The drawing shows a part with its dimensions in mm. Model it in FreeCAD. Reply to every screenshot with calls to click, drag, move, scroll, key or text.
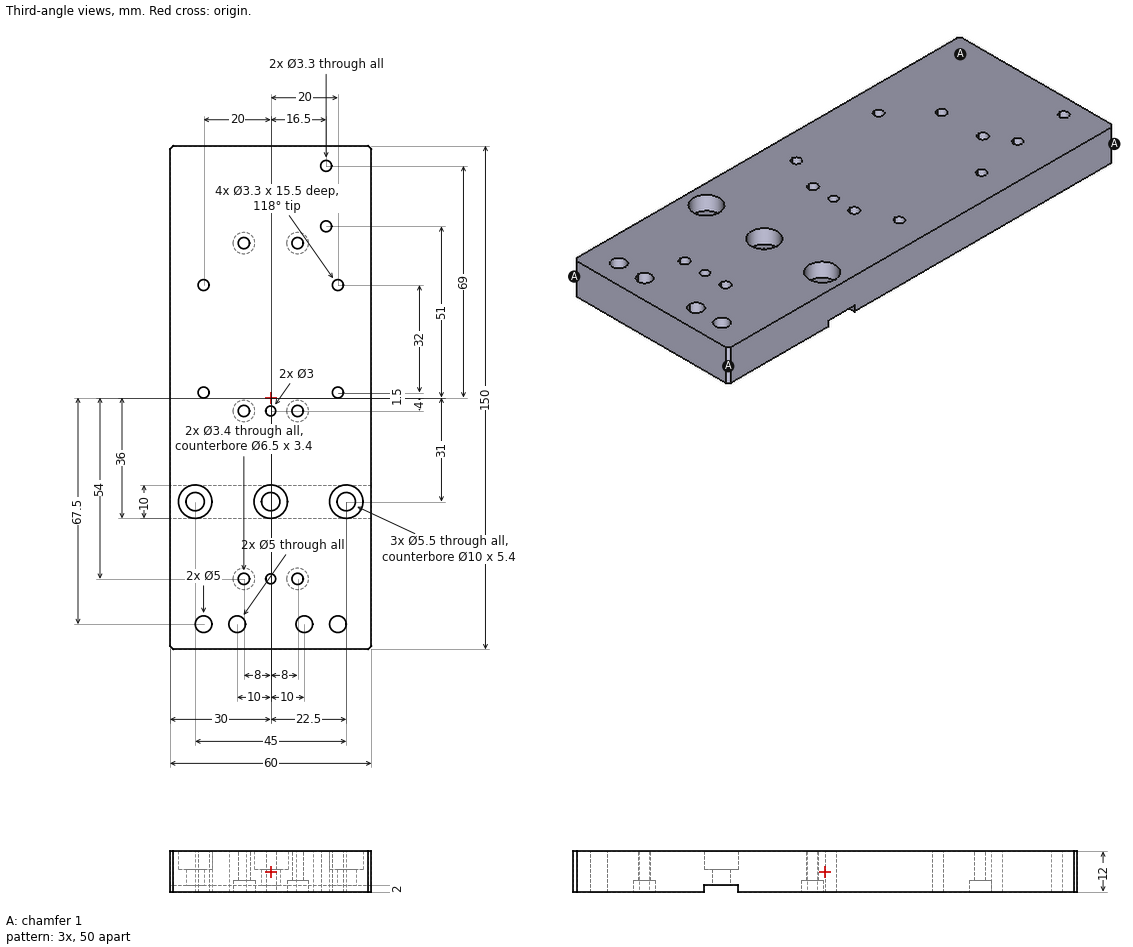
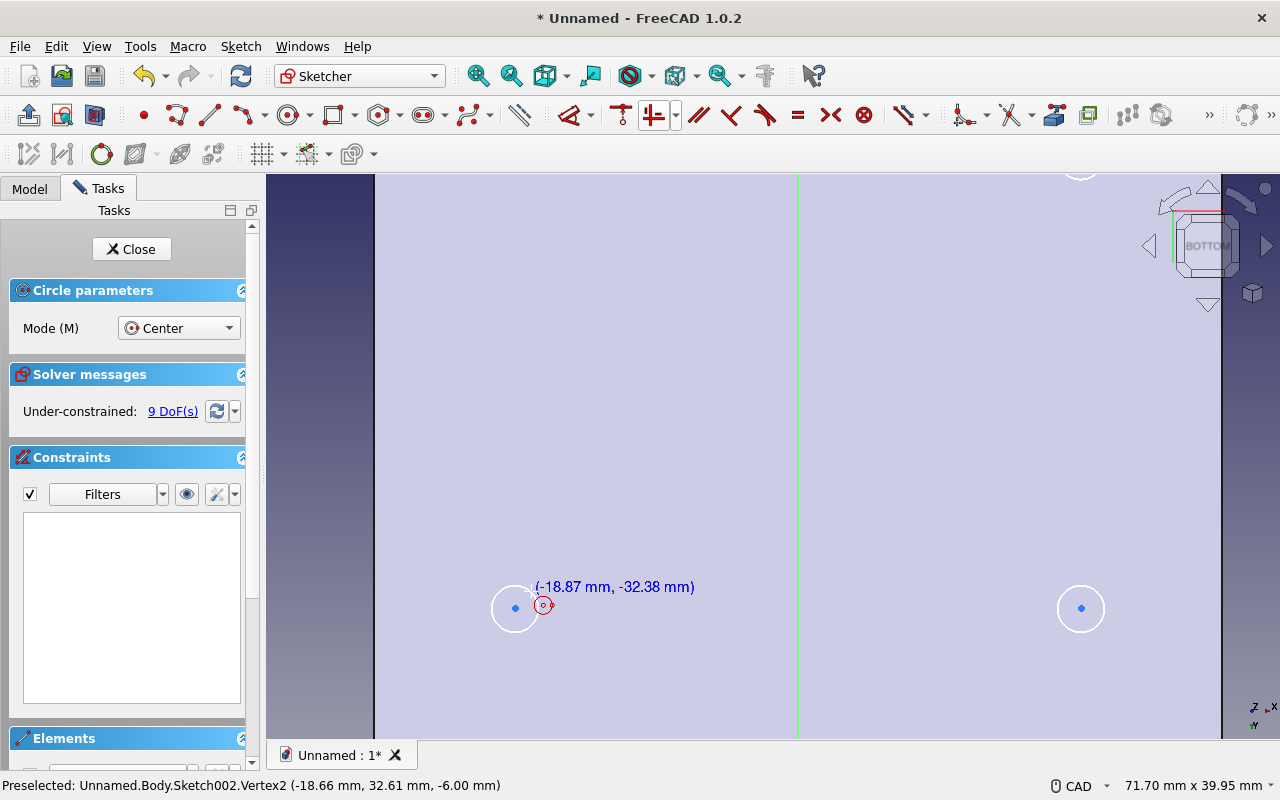
scroll(515, 609, down, 2)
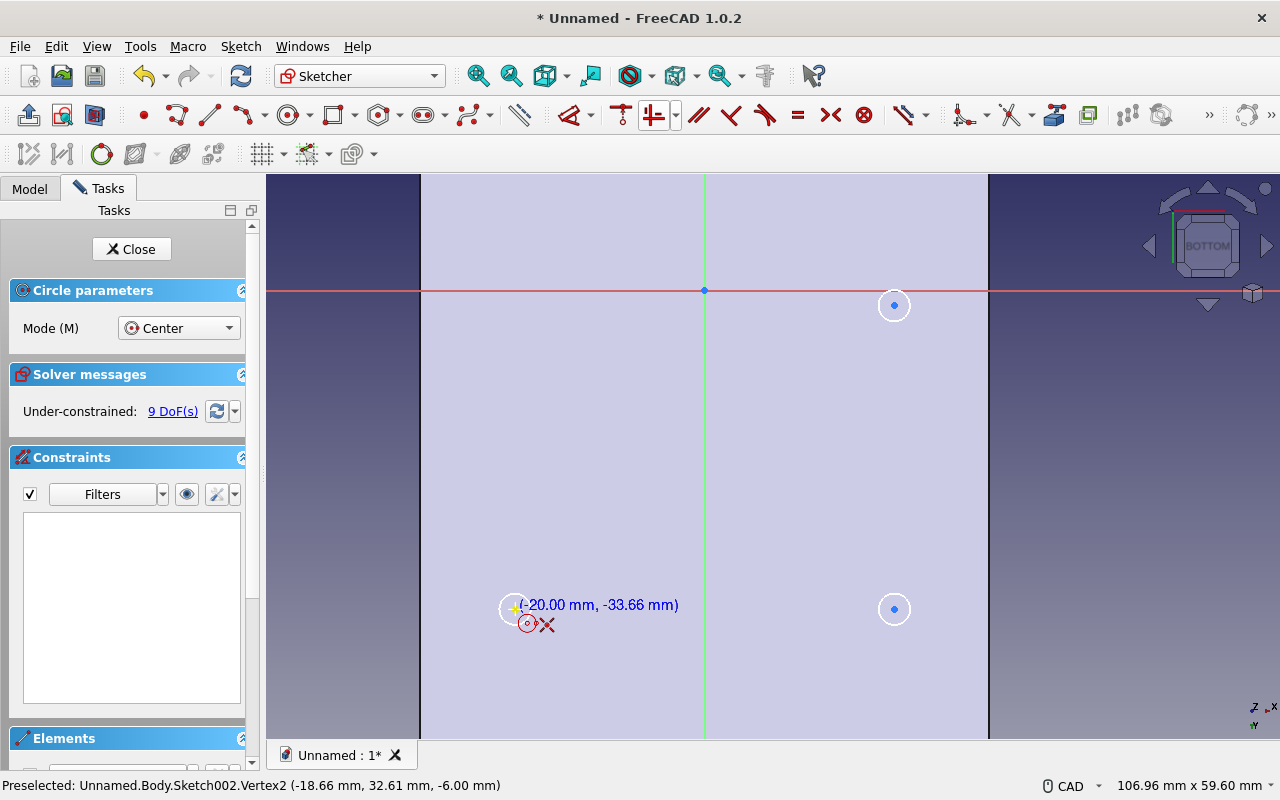
scroll(515, 305, up, 2)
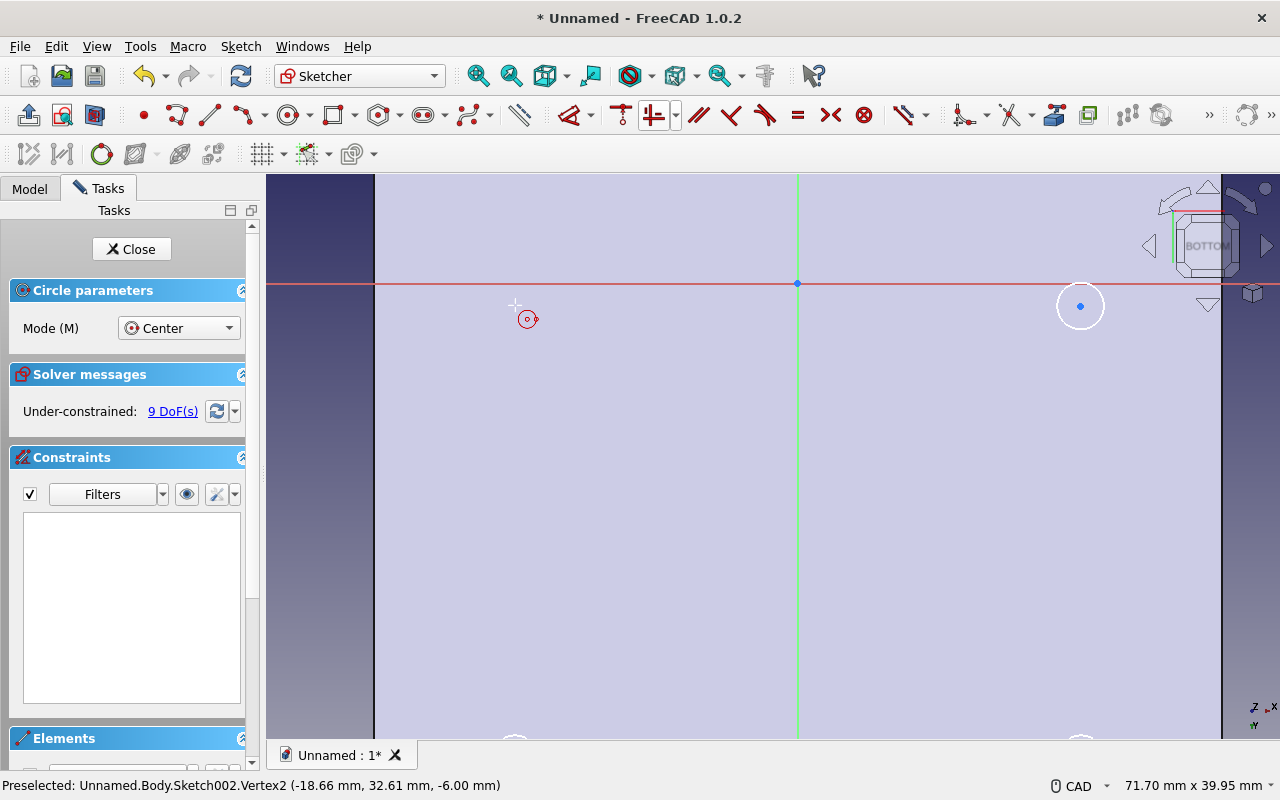
click(515, 305)
click(531, 321)
key(Escape)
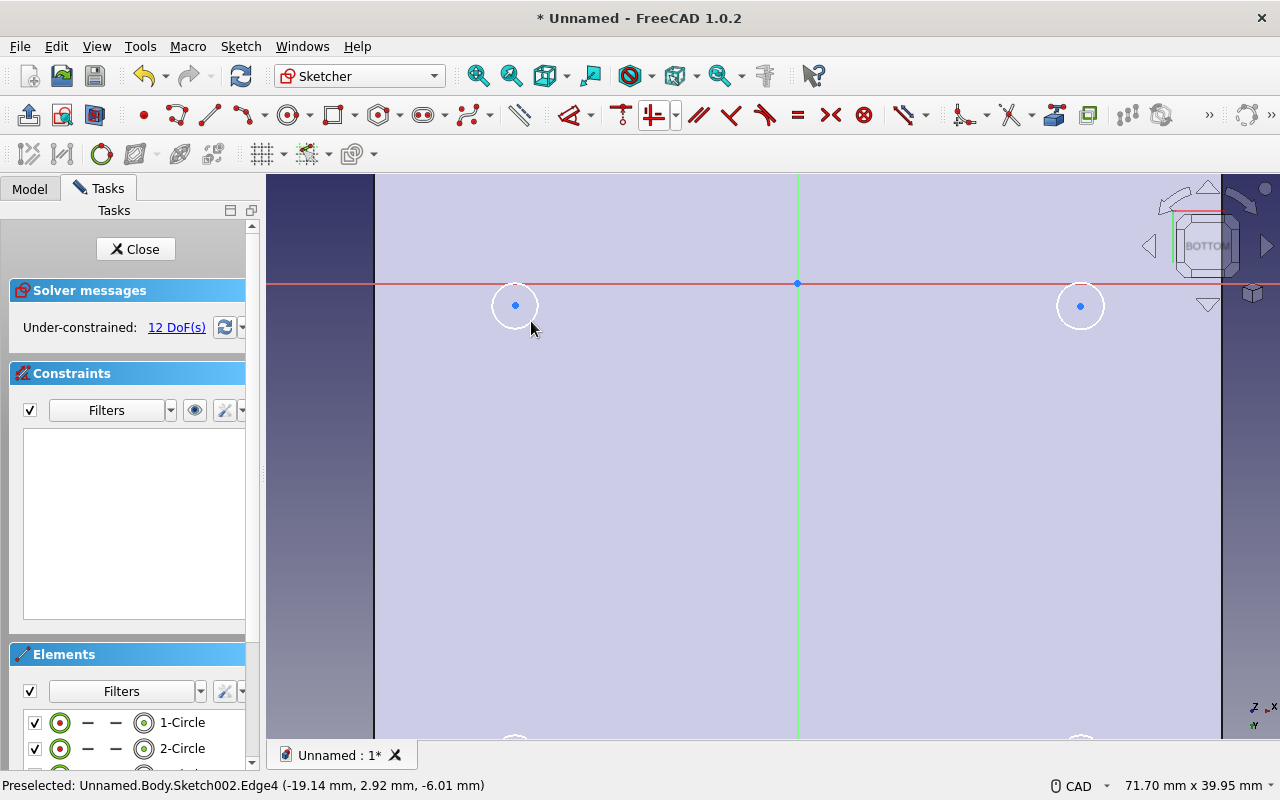
scroll(515, 304, down, 2)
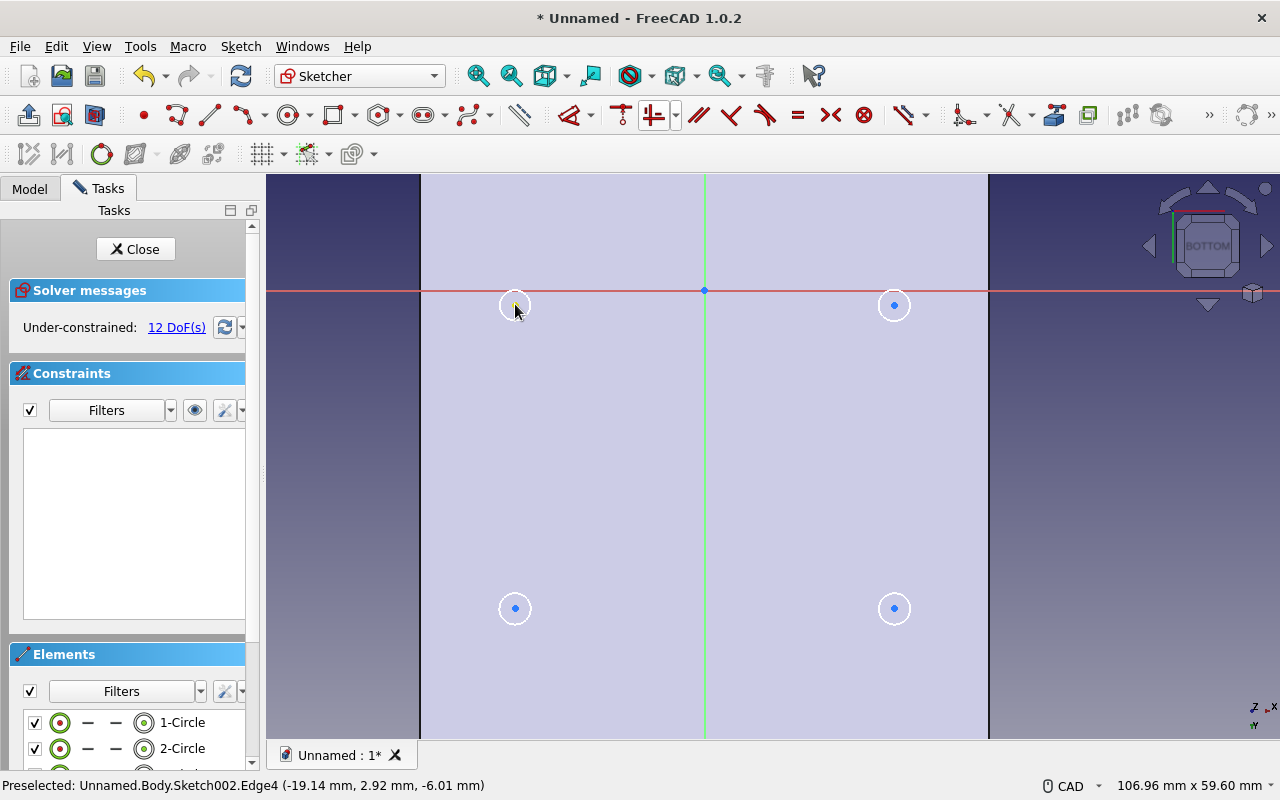
click(906, 598)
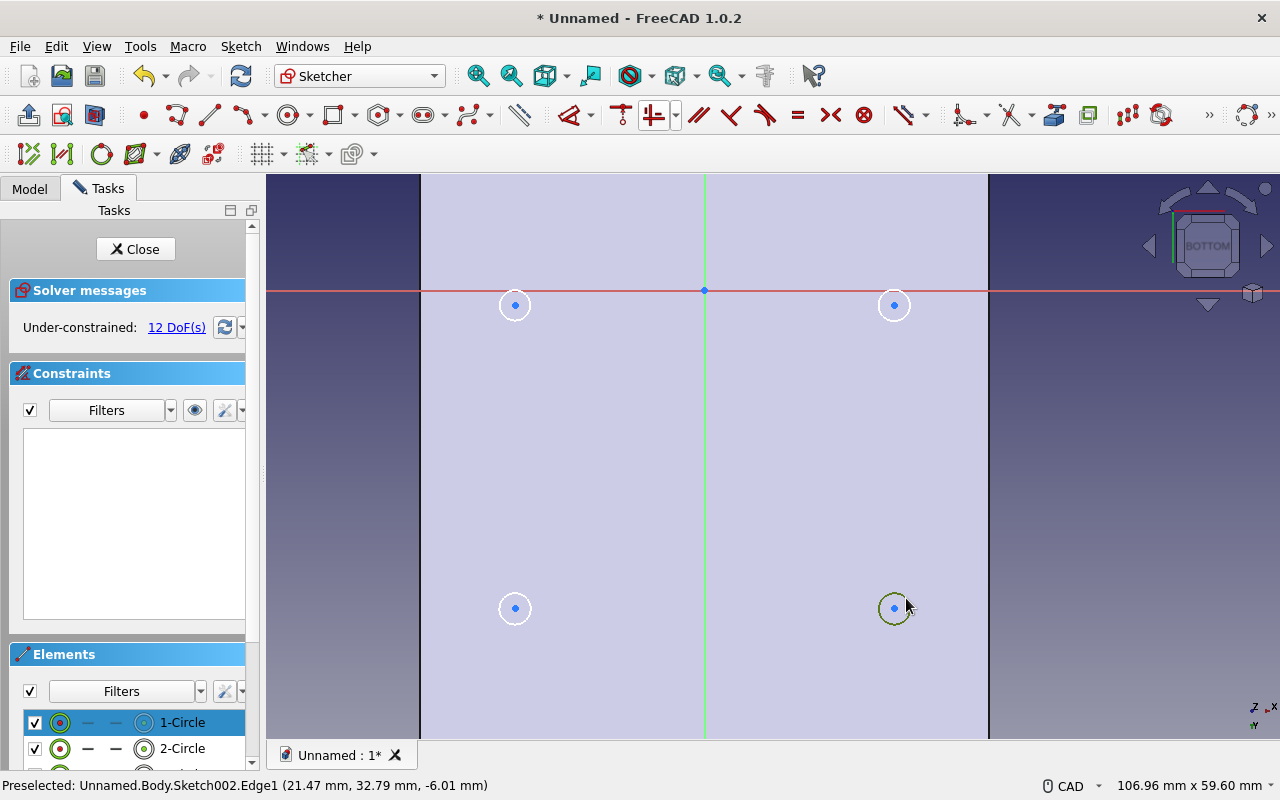
click(905, 294)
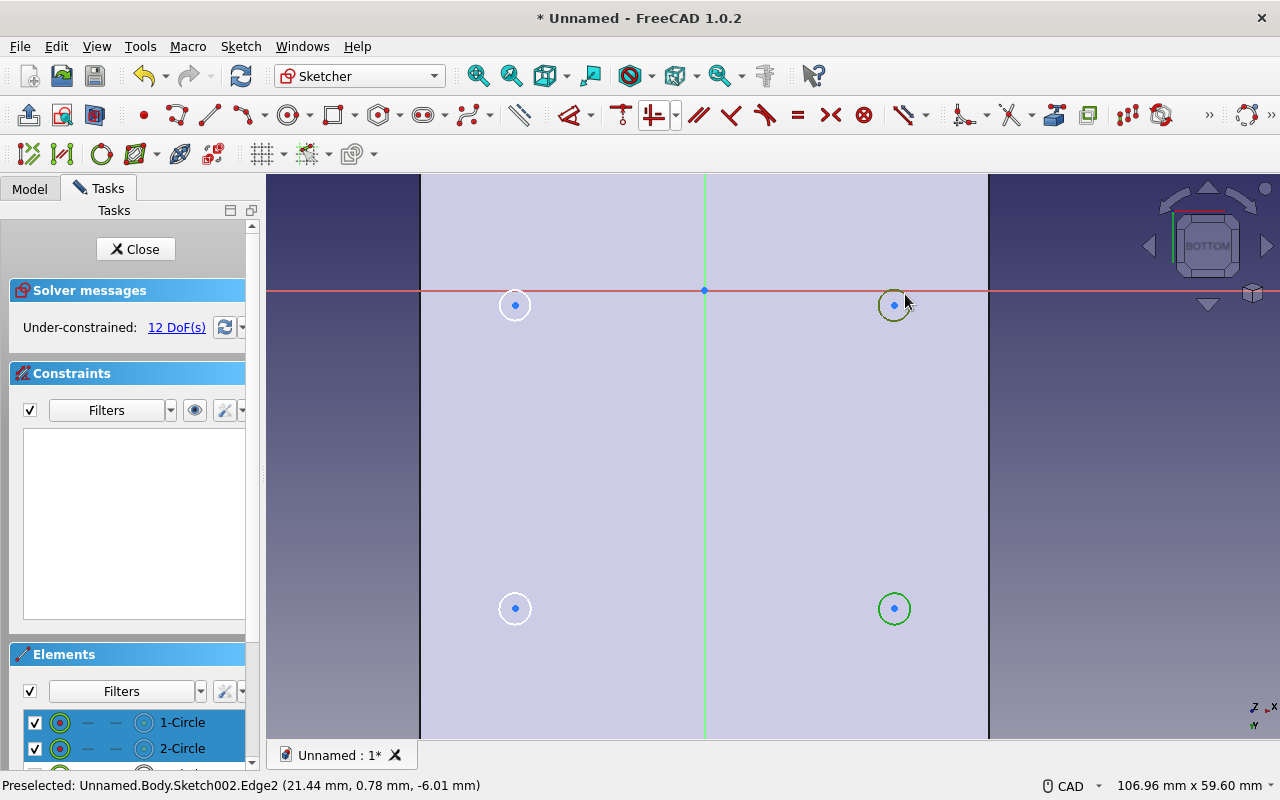
click(526, 598)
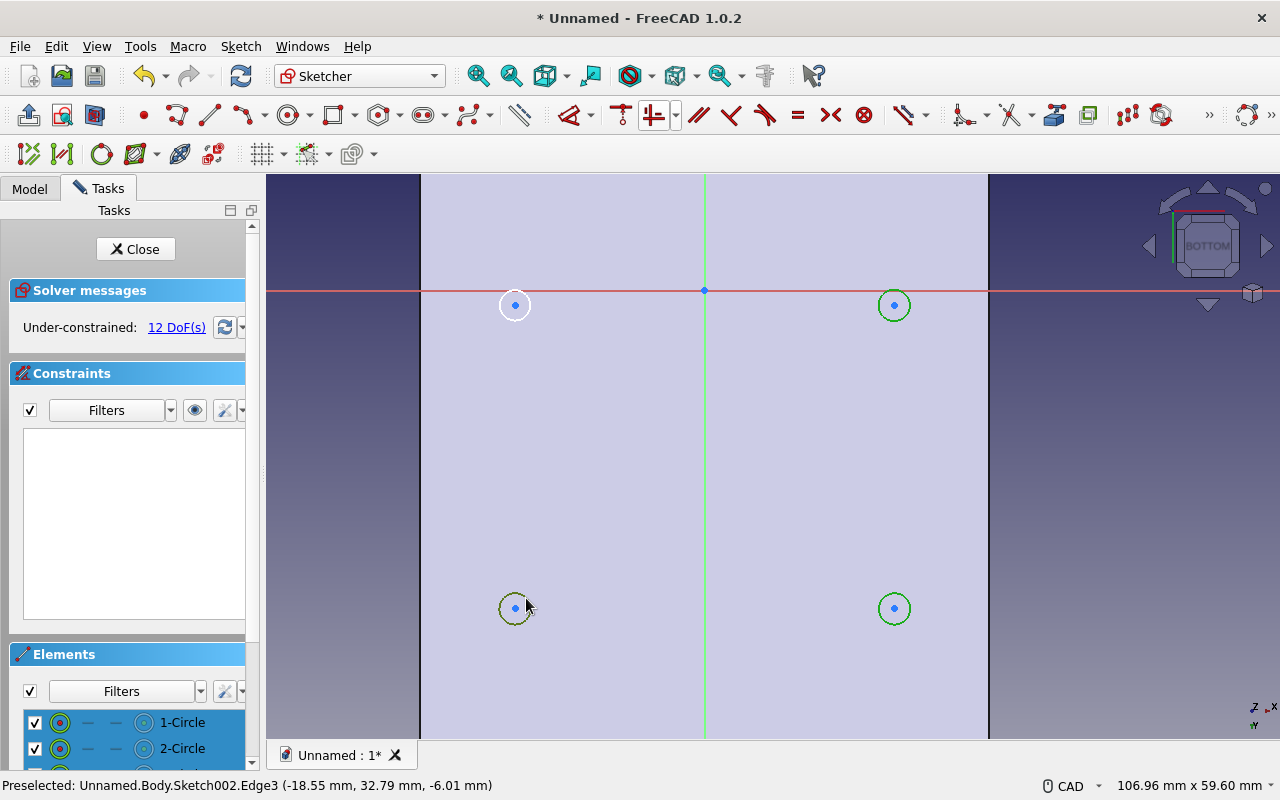
click(504, 316)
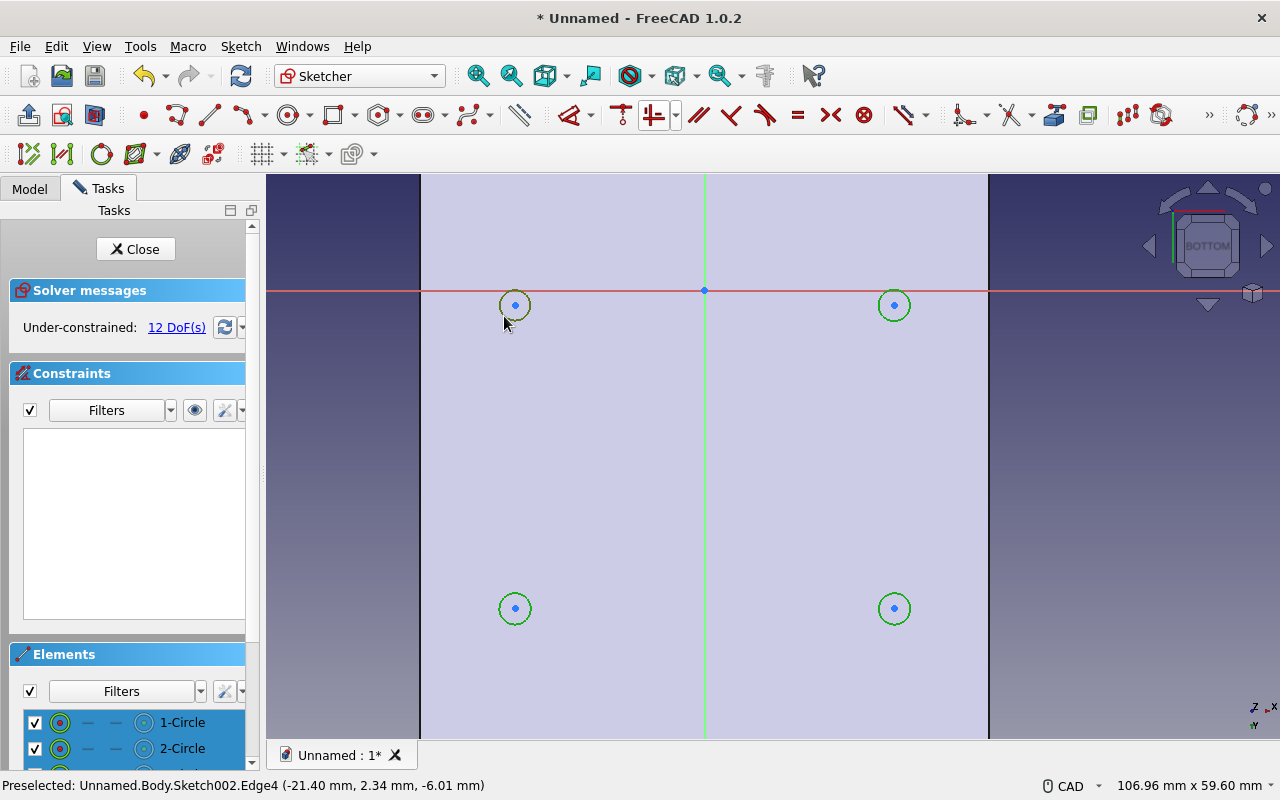
click(798, 116)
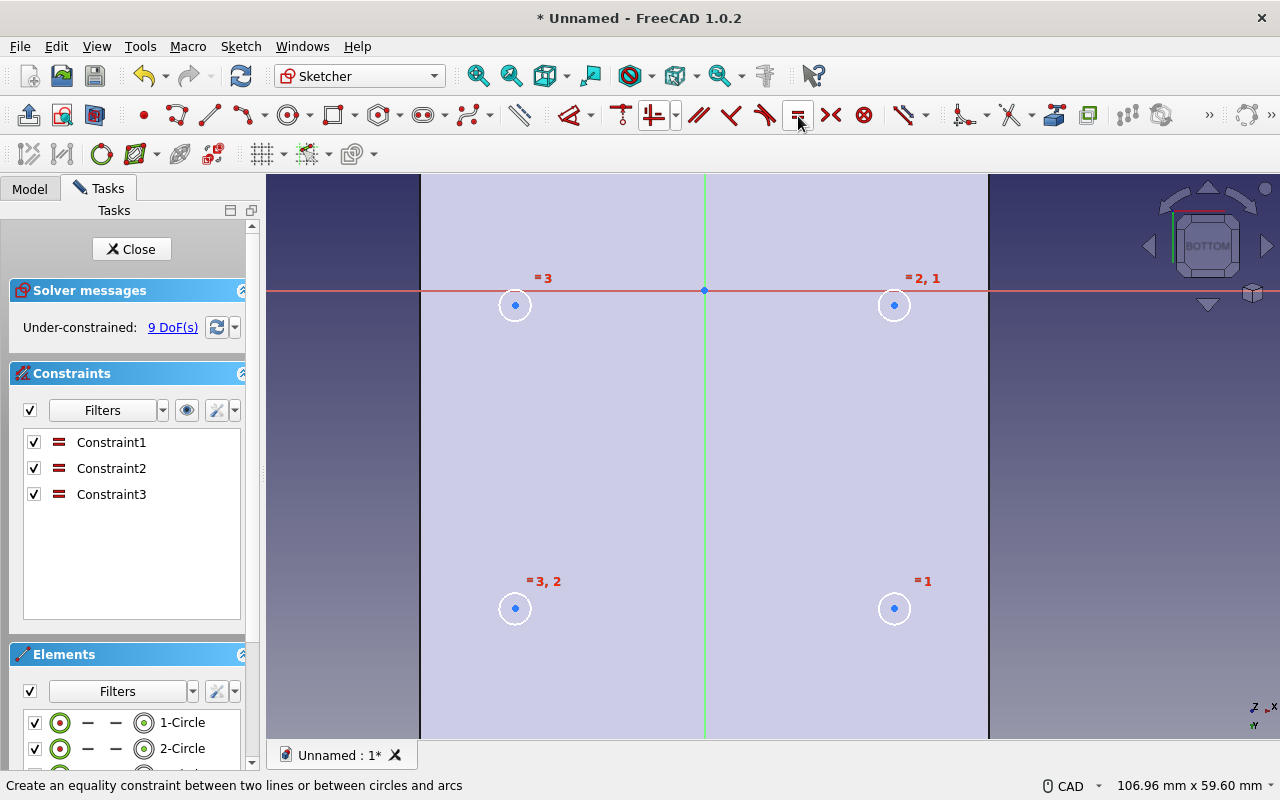
click(895, 609)